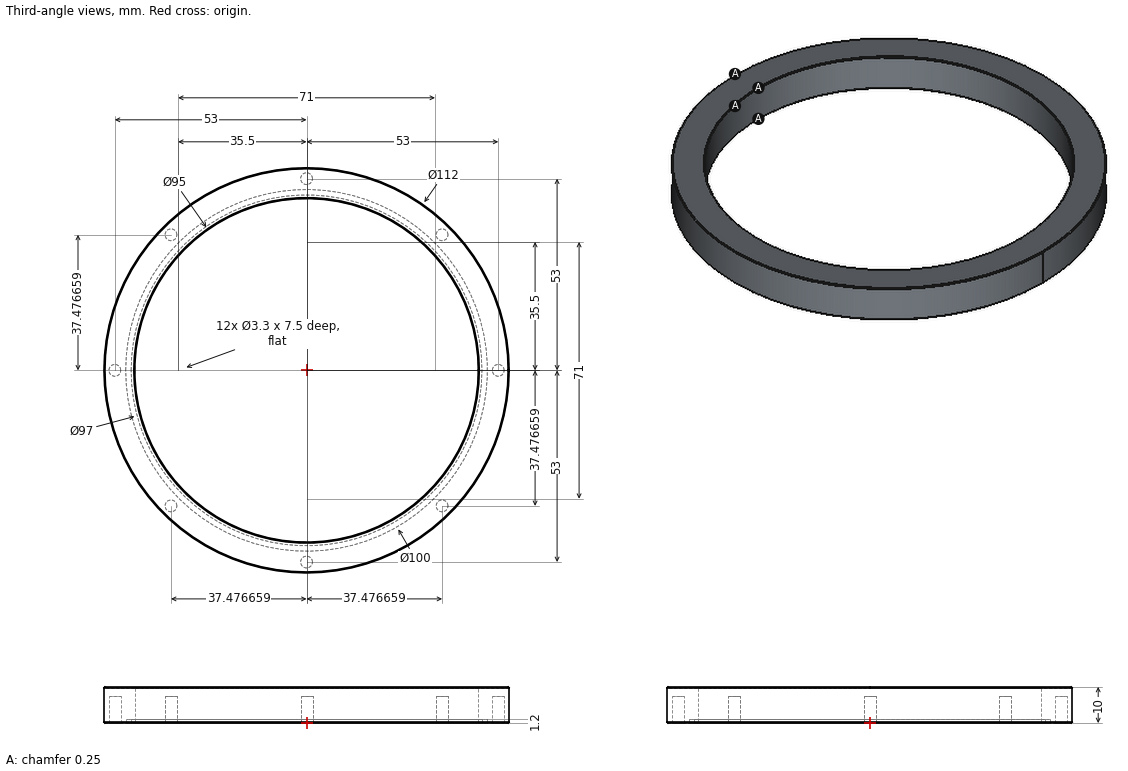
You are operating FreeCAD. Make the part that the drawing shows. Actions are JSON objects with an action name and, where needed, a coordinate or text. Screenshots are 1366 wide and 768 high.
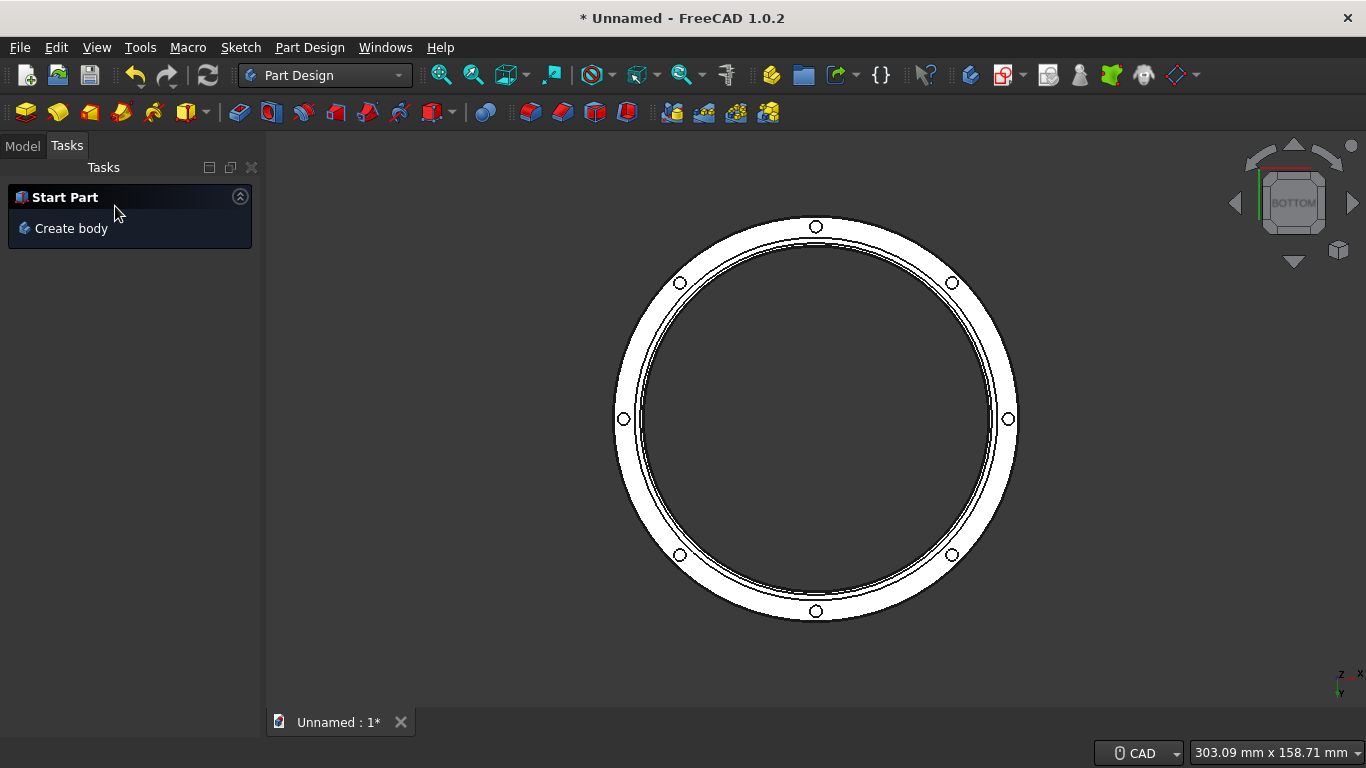
{"action": "key", "text": "0"}